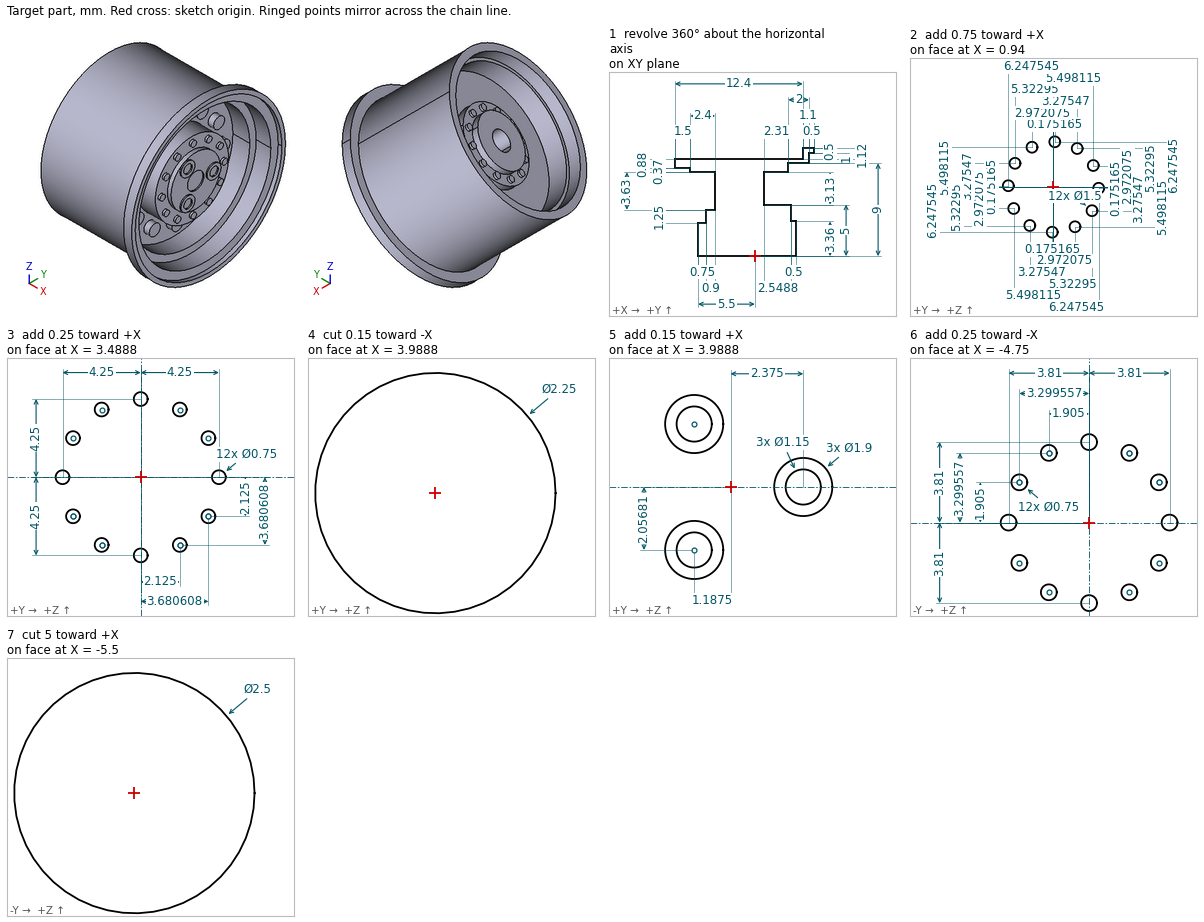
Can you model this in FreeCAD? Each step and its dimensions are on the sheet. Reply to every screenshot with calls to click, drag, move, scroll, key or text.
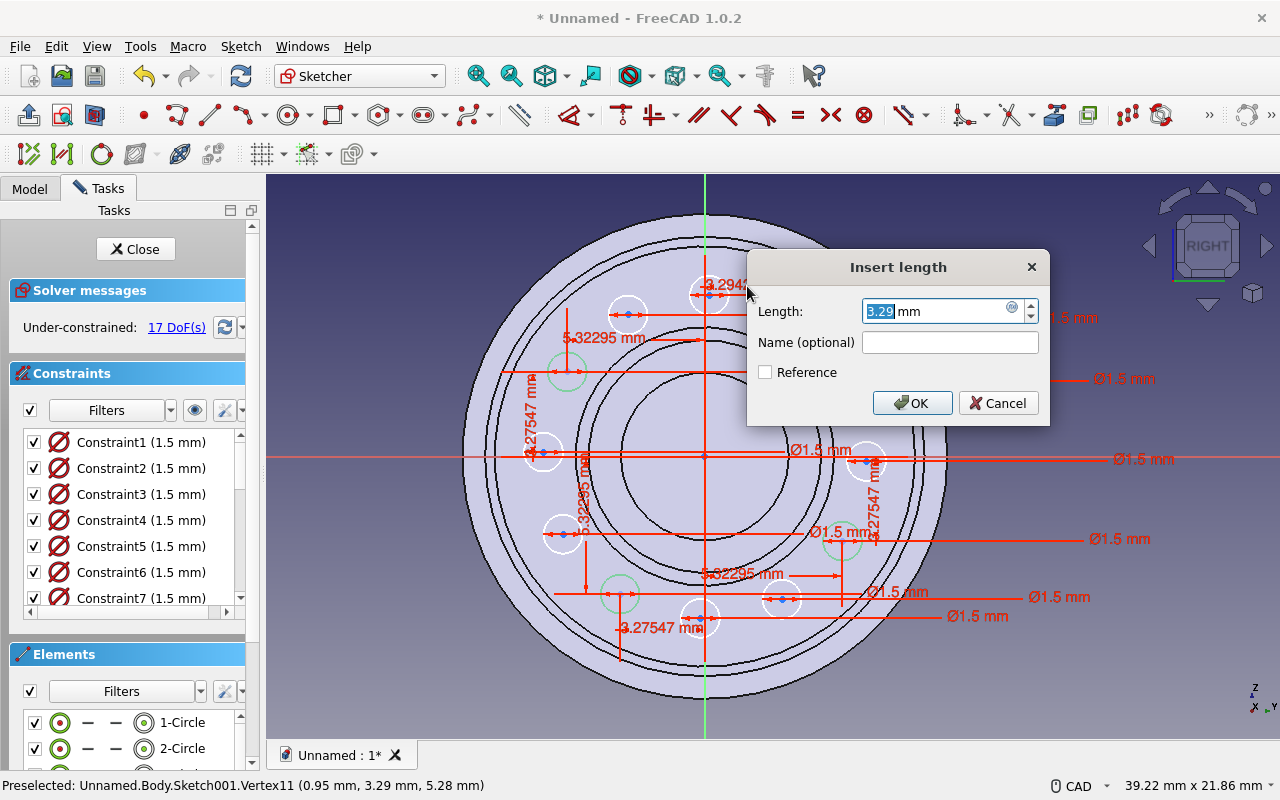
text(3.27547)
key(Return)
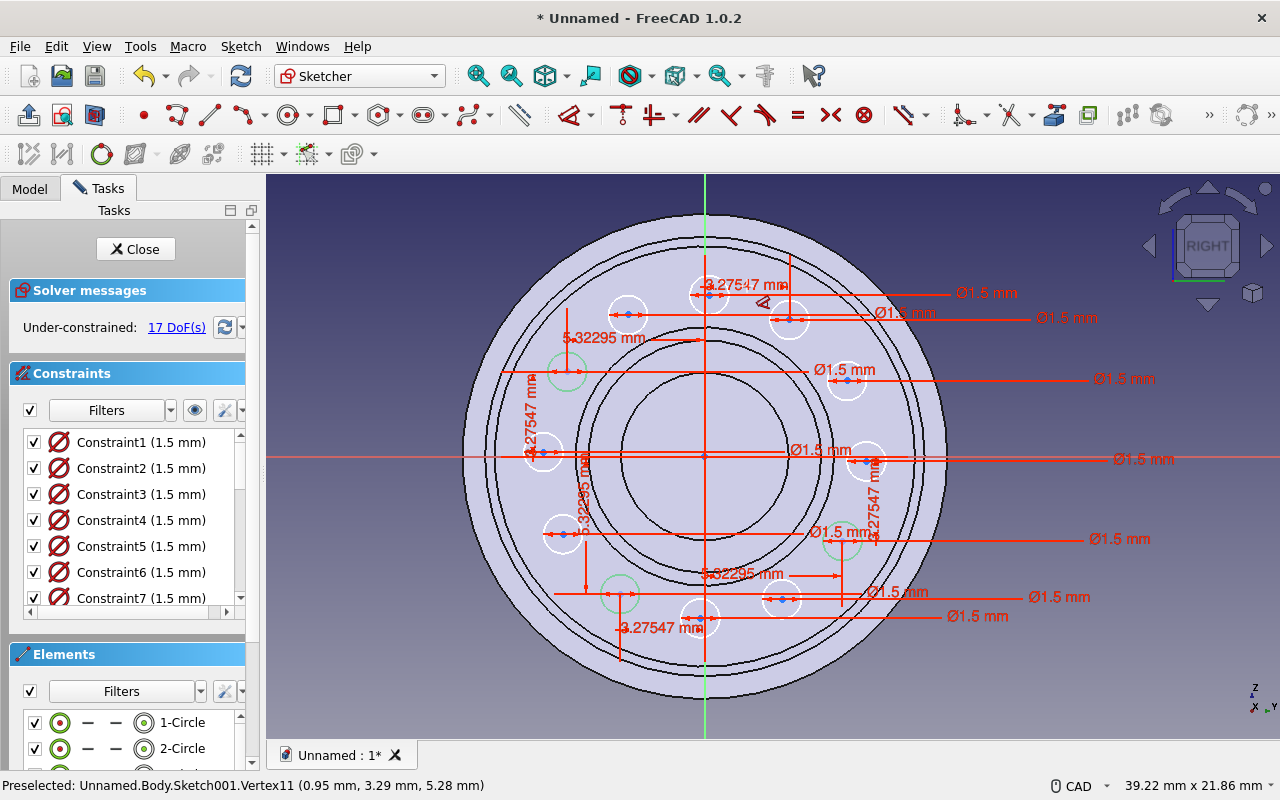
click(790, 320)
click(824, 357)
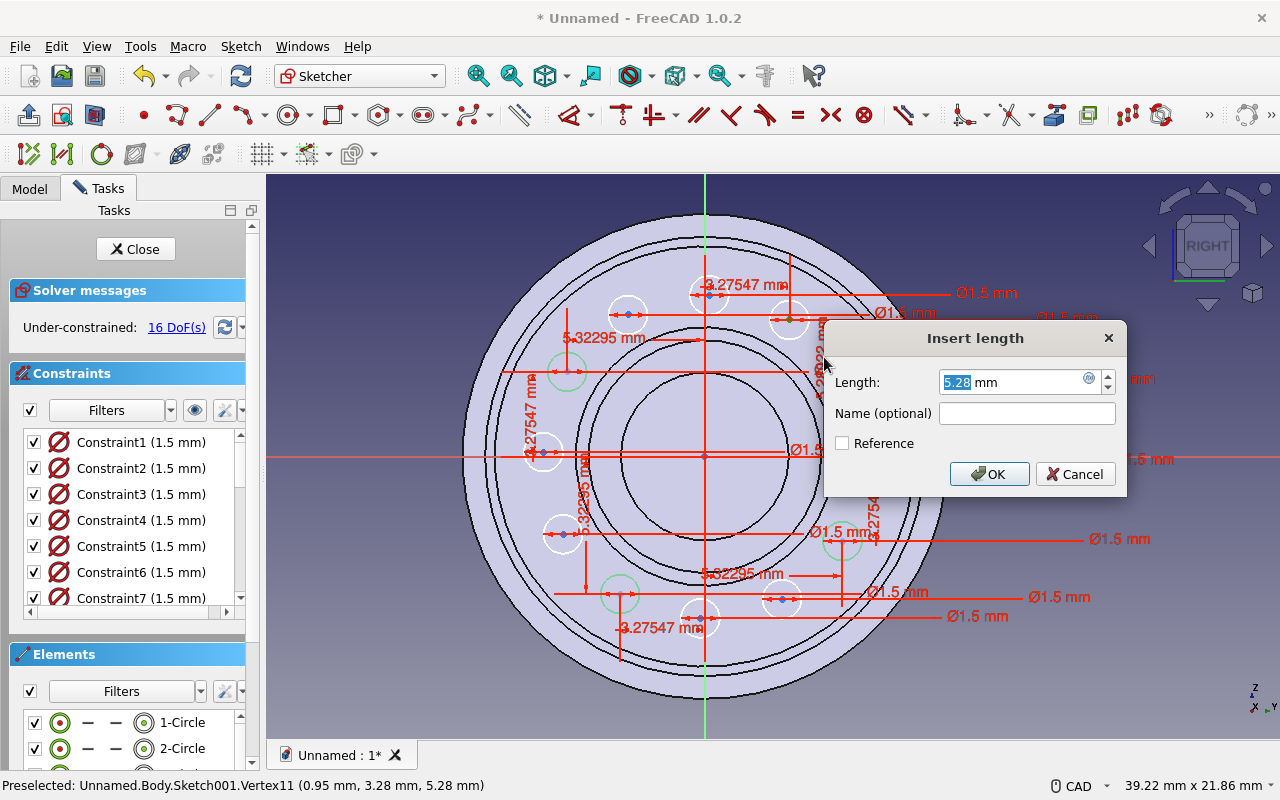
text(5.32295)
key(Return)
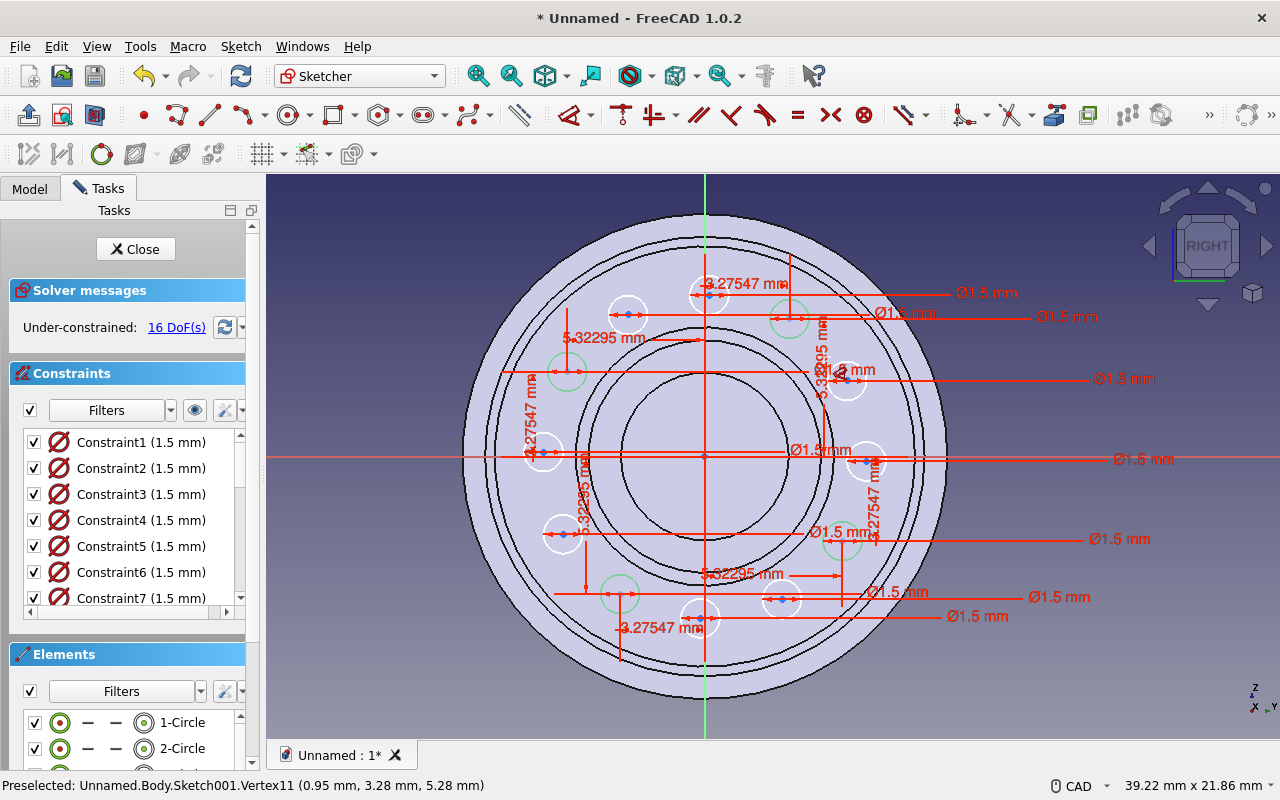
click(866, 461)
click(786, 495)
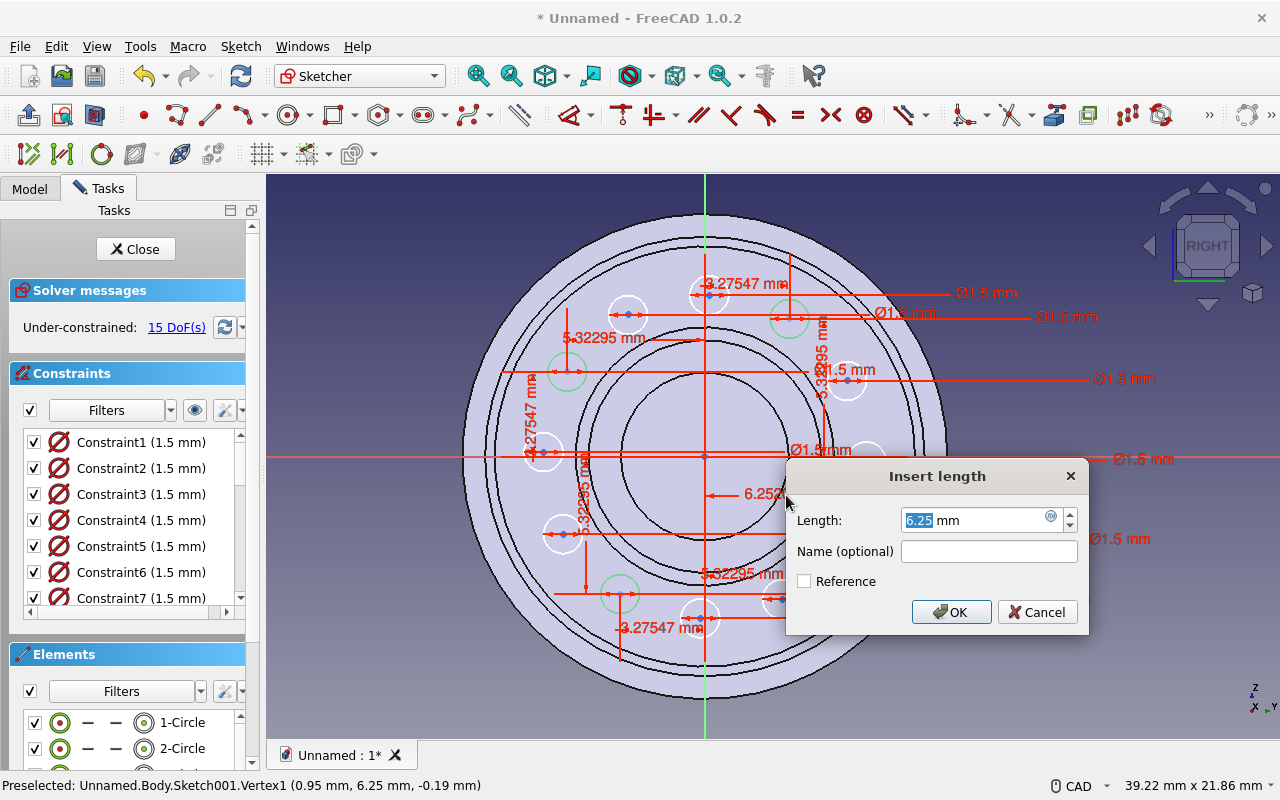
text(6.247545)
key(Return)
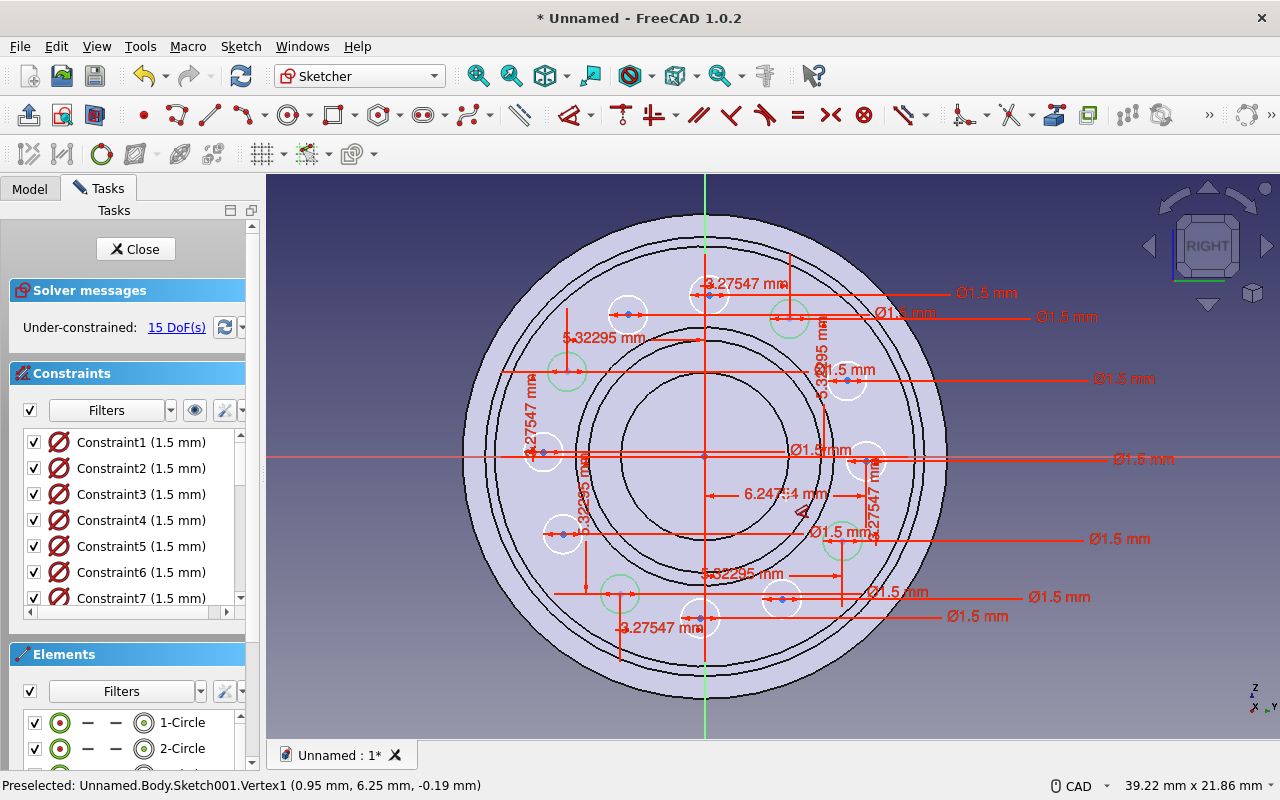
scroll(866, 461, up, 11)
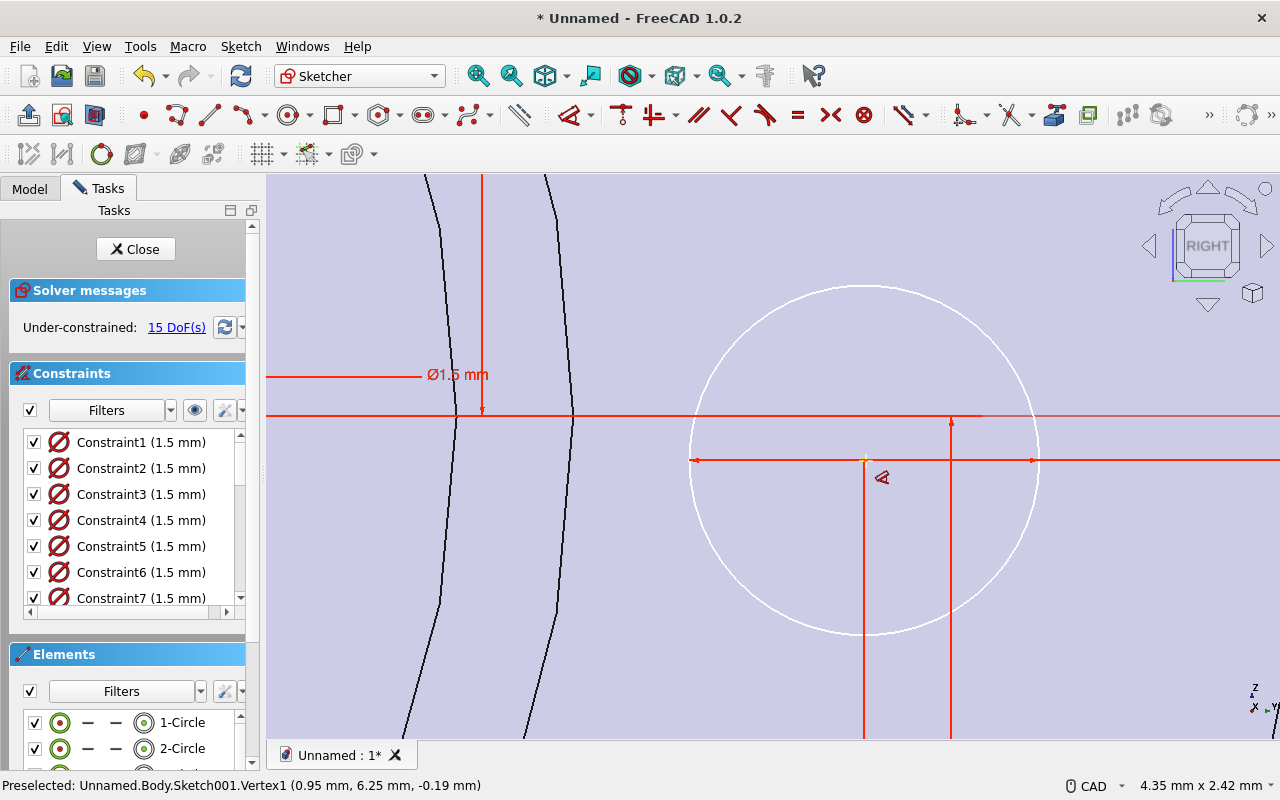
click(864, 460)
click(898, 438)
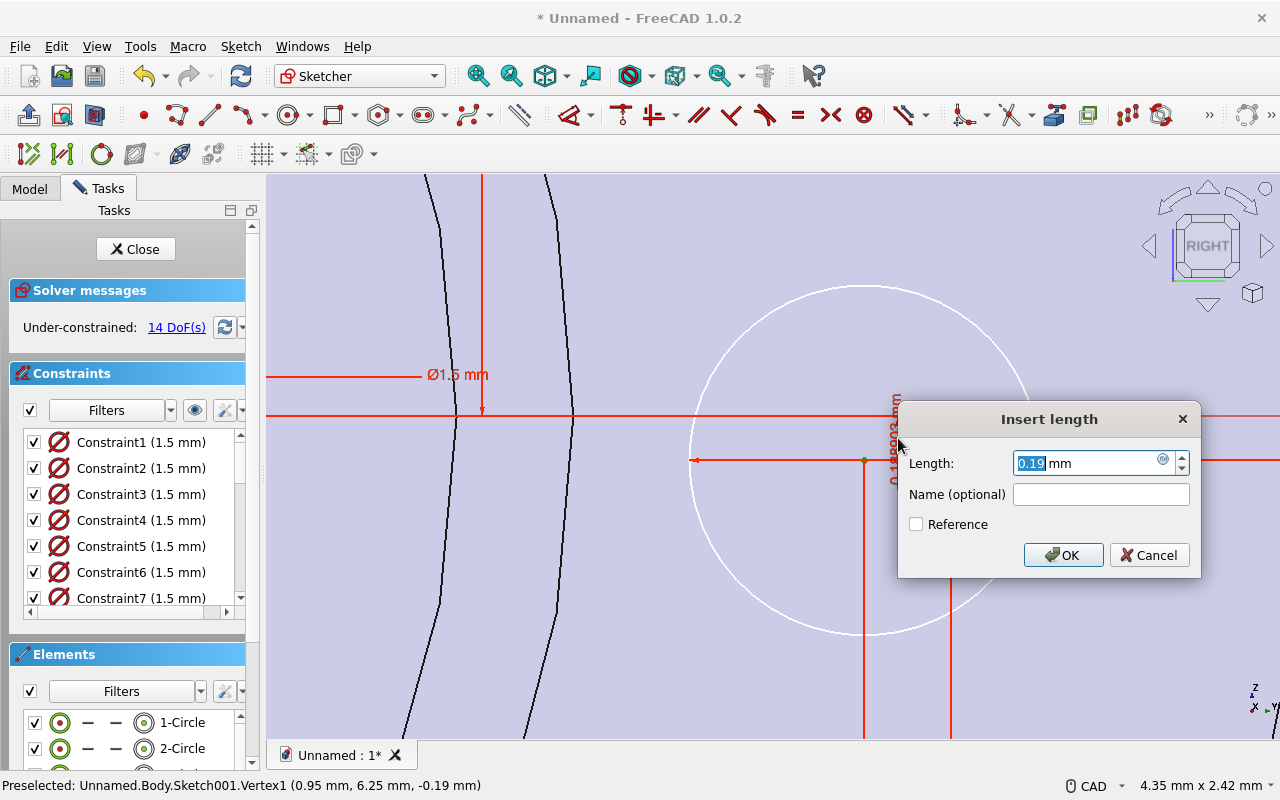
text(0.175165)
key(Return)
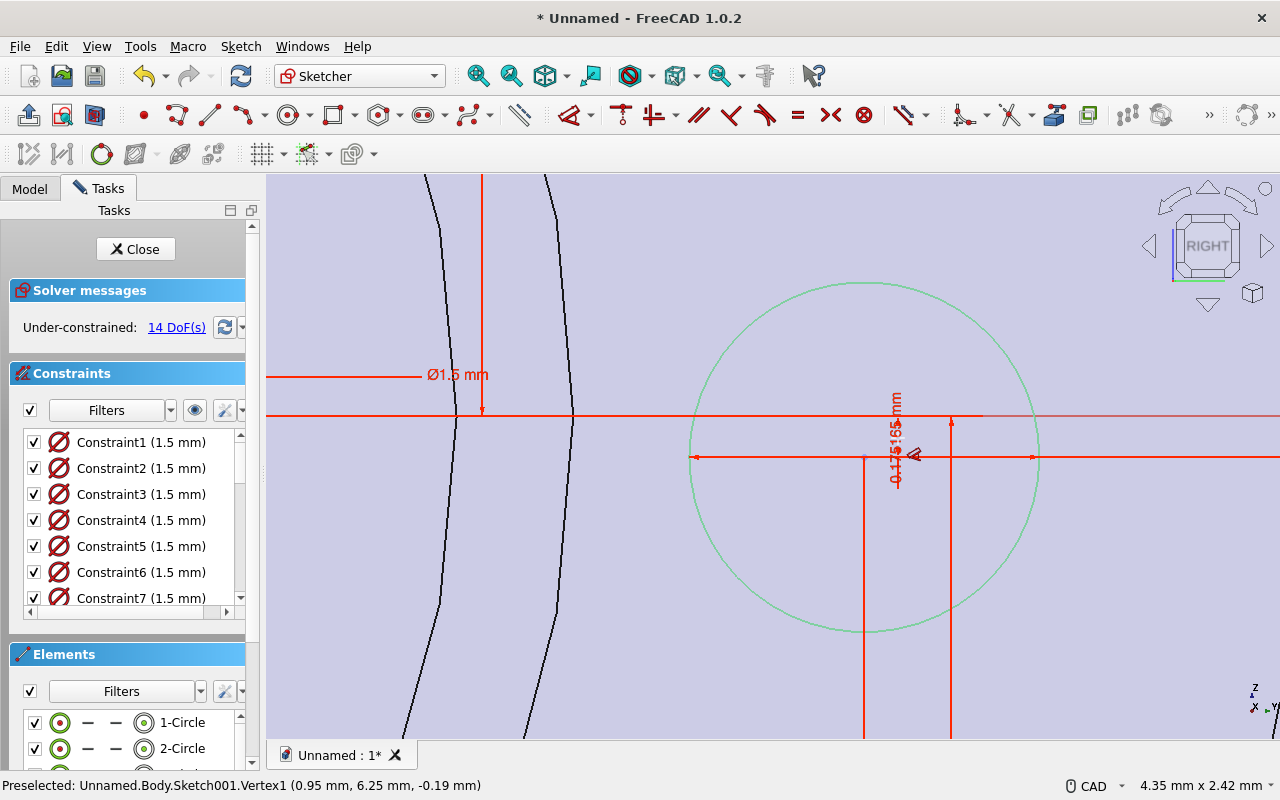
scroll(866, 462, down, 11)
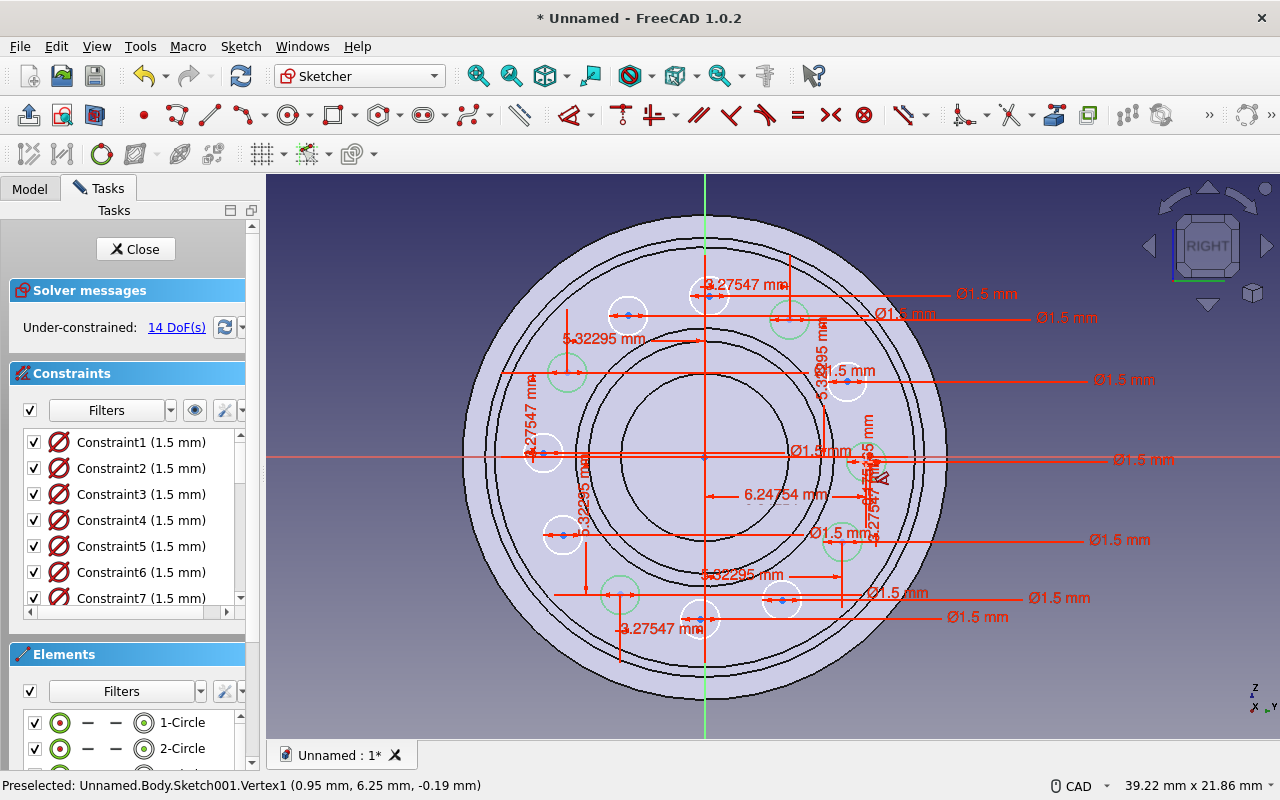
click(782, 600)
click(743, 634)